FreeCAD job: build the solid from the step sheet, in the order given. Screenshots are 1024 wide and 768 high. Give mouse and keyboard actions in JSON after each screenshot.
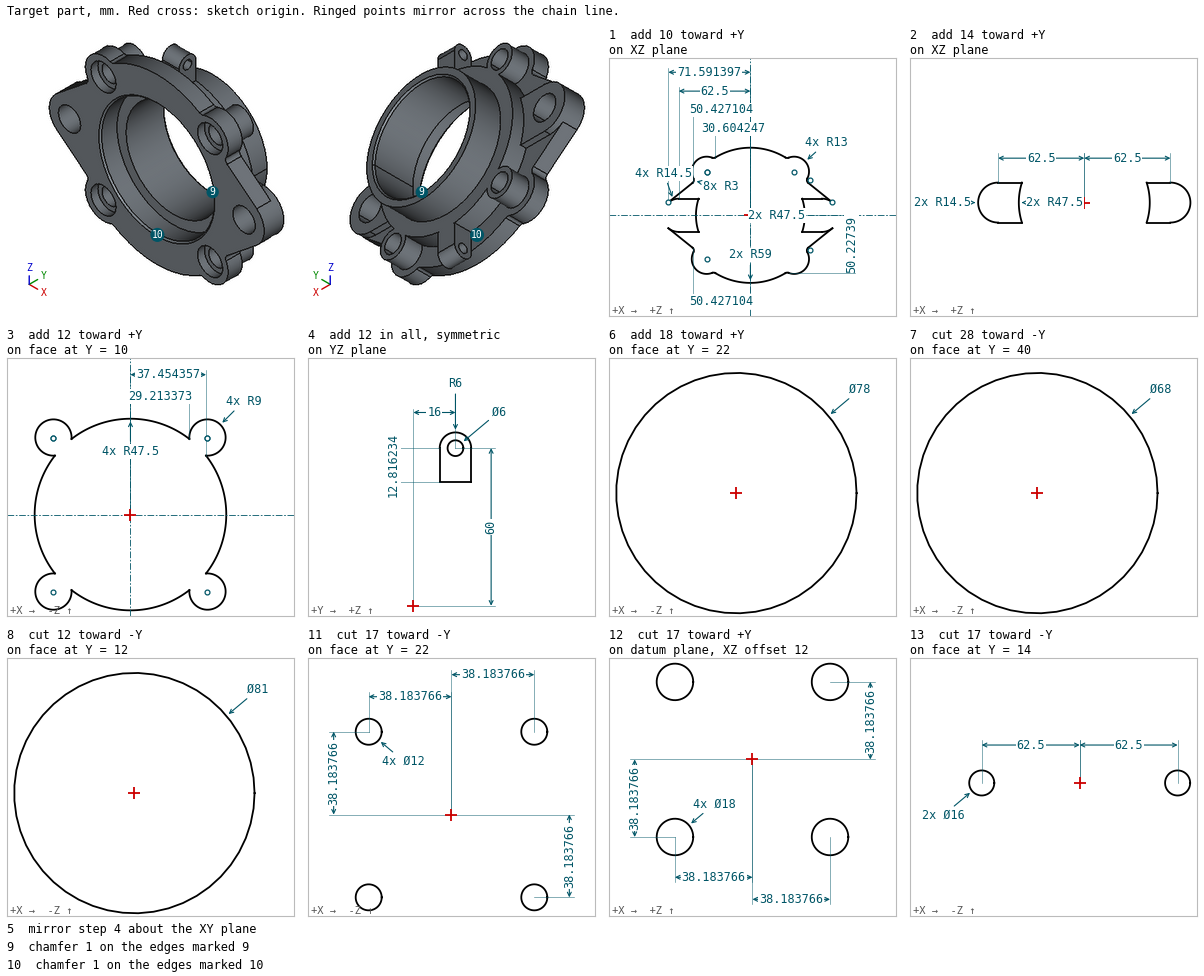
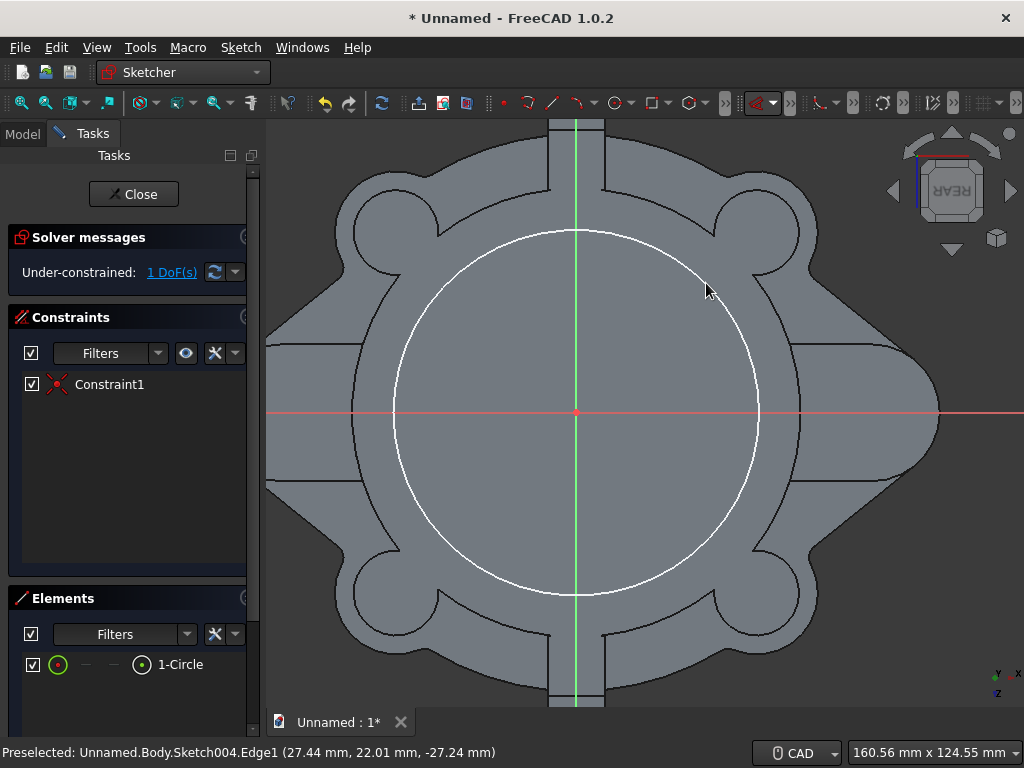
{"action": "key", "text": "d"}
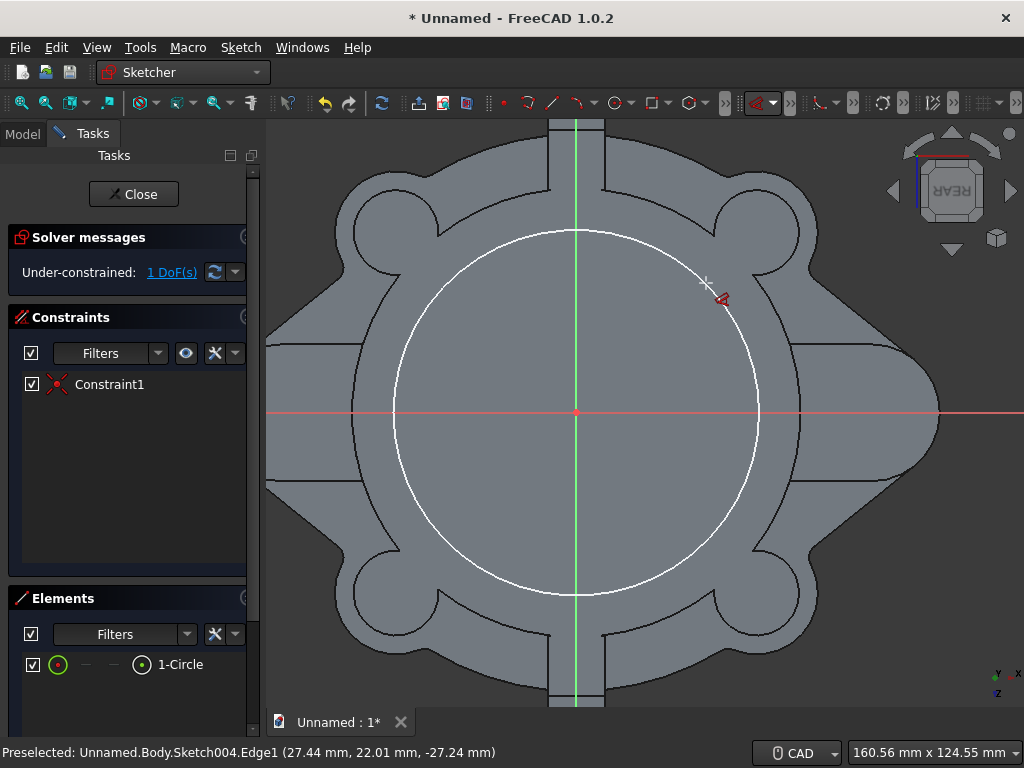
{"action": "left_click", "coordinate": [705, 283]}
{"action": "left_click", "coordinate": [728, 260]}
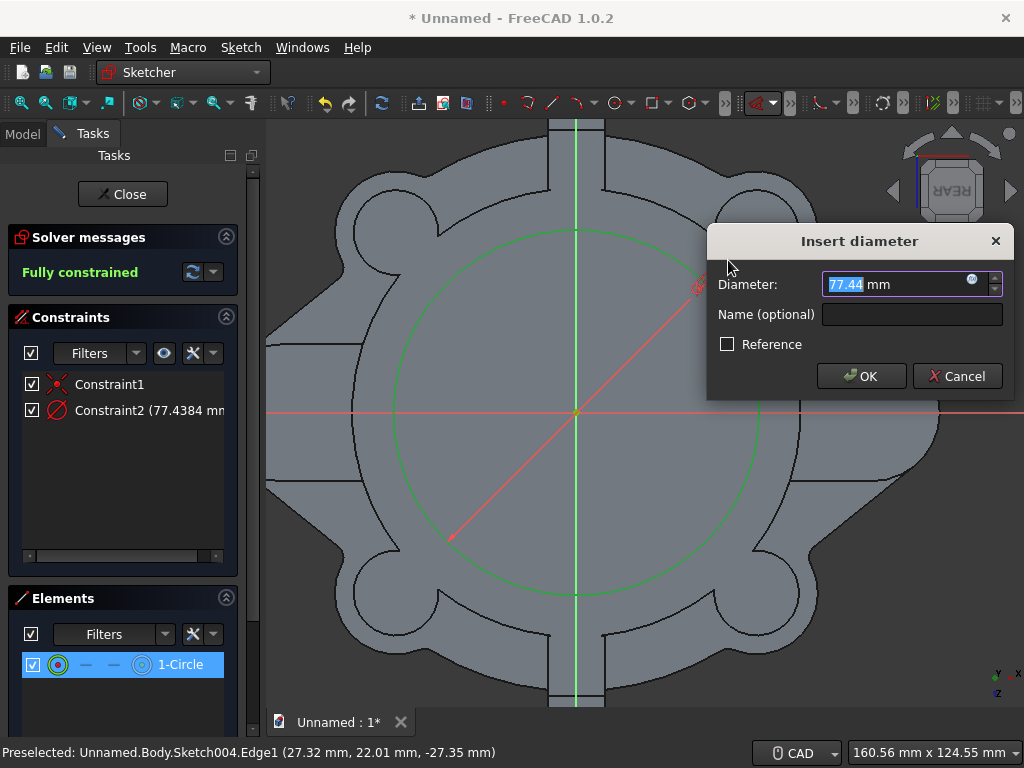
{"action": "type", "text": "78"}
{"action": "key", "text": "Return"}
{"action": "key", "text": "Escape"}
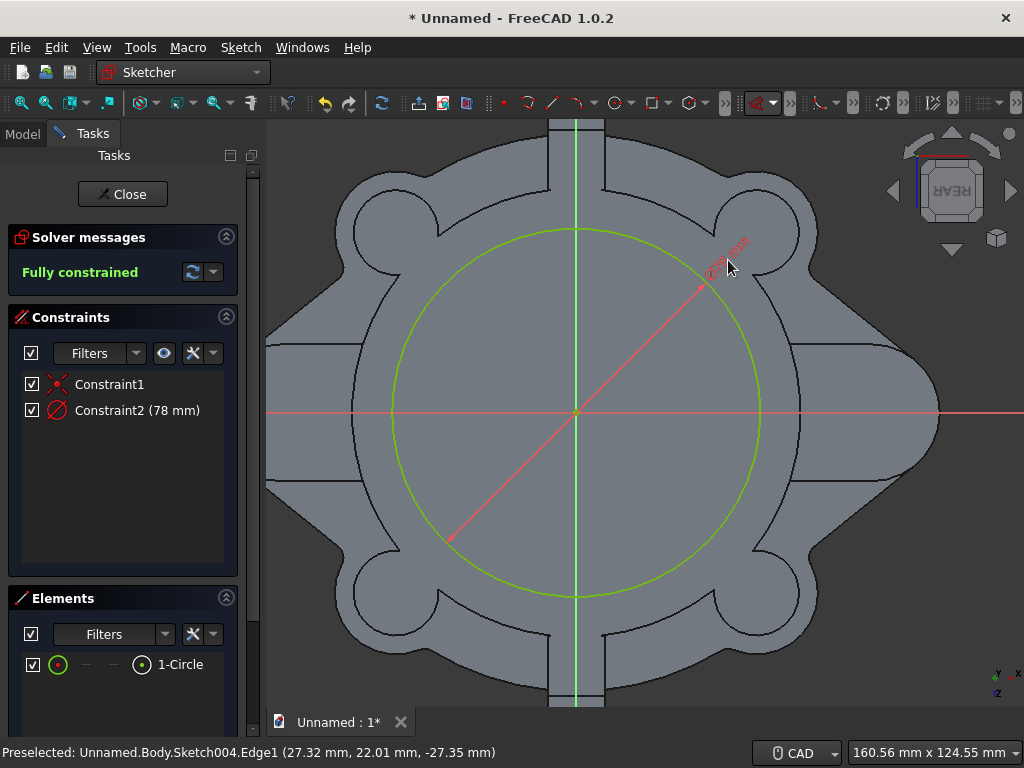
{"action": "left_click", "coordinate": [123, 194]}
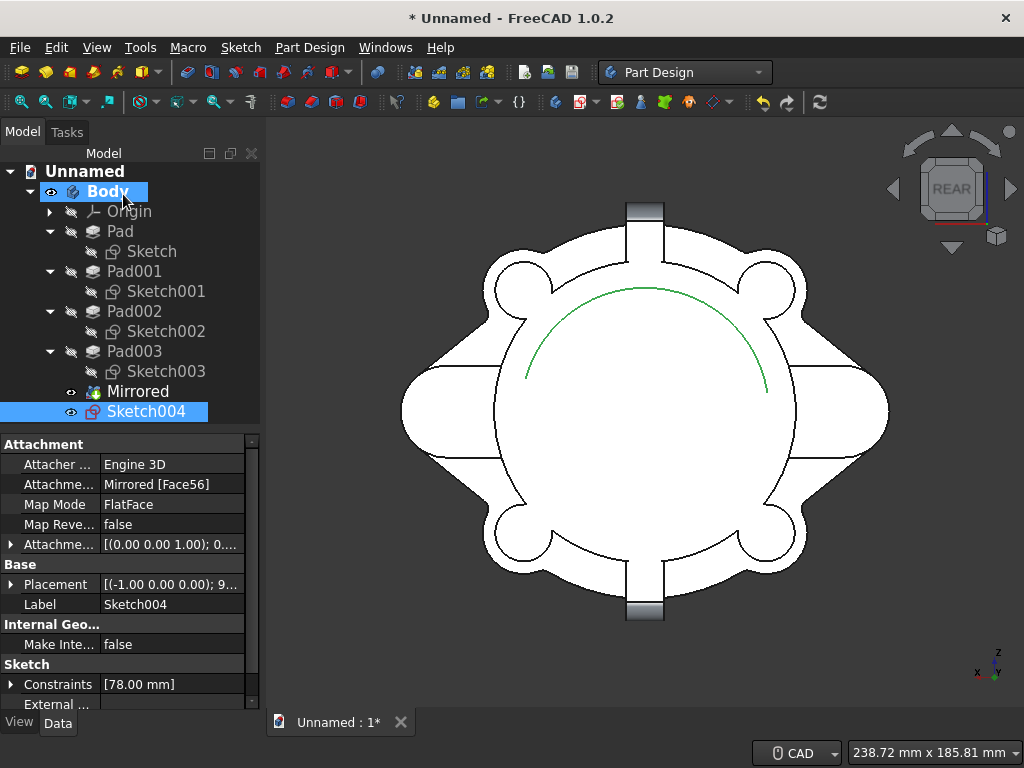
{"action": "left_click", "coordinate": [22, 72]}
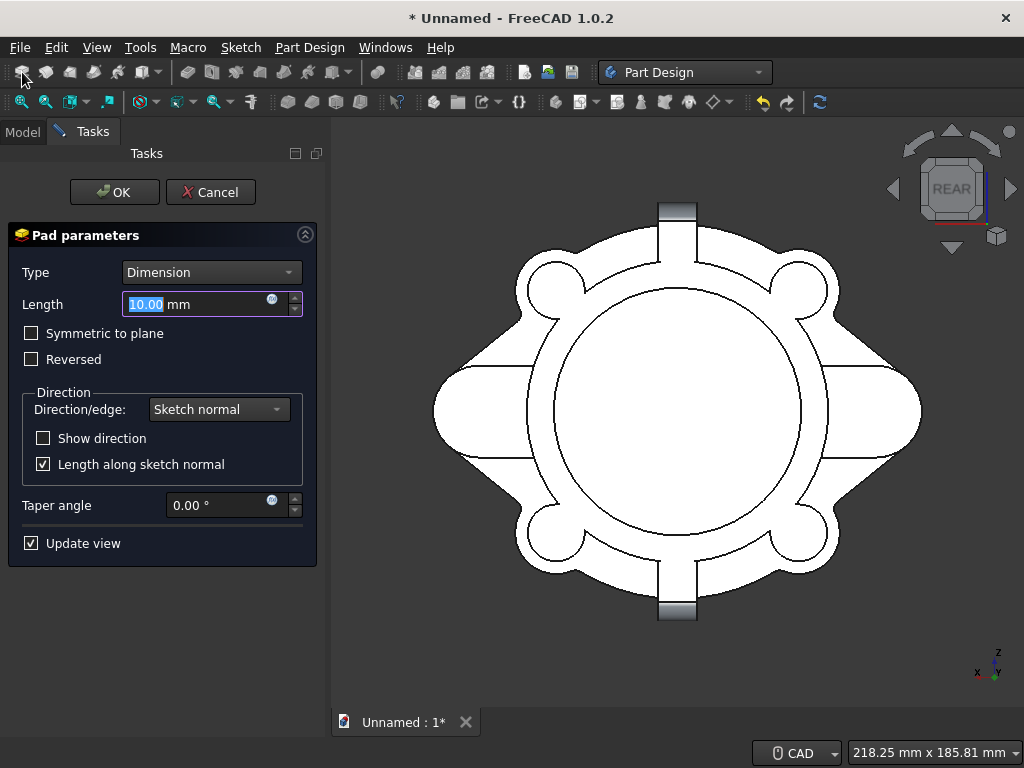
{"action": "type", "text": "18"}
{"action": "key", "text": "Tab"}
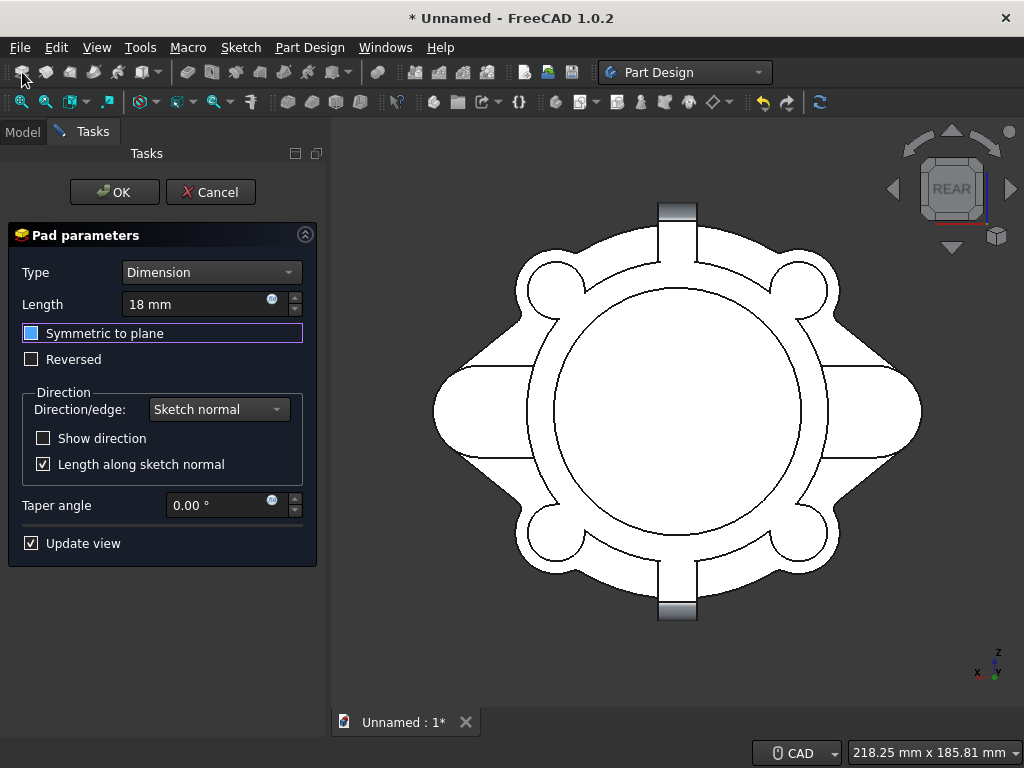
{"action": "left_click", "coordinate": [115, 192]}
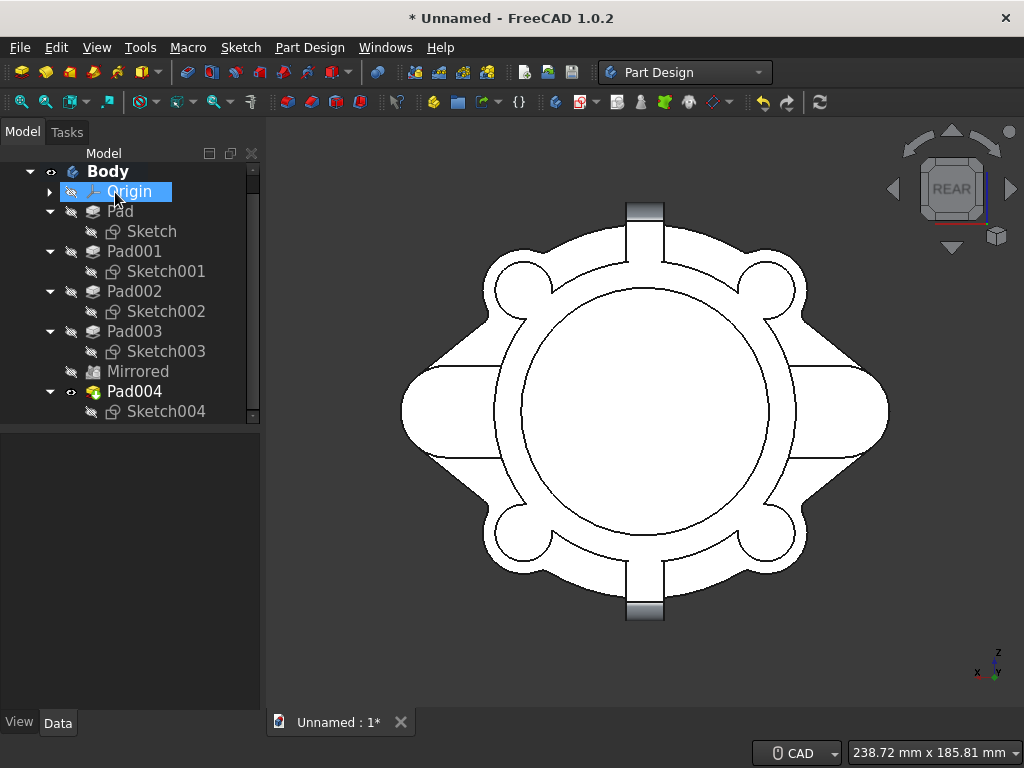
{"action": "left_click", "coordinate": [645, 411]}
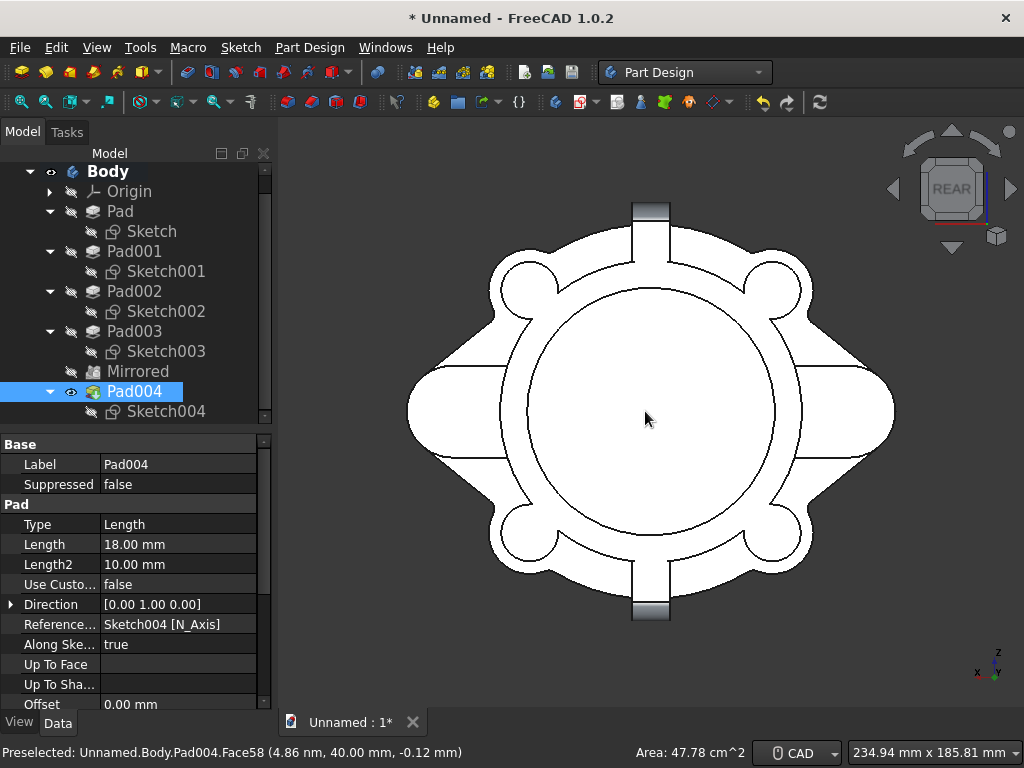
{"action": "left_click", "coordinate": [580, 102]}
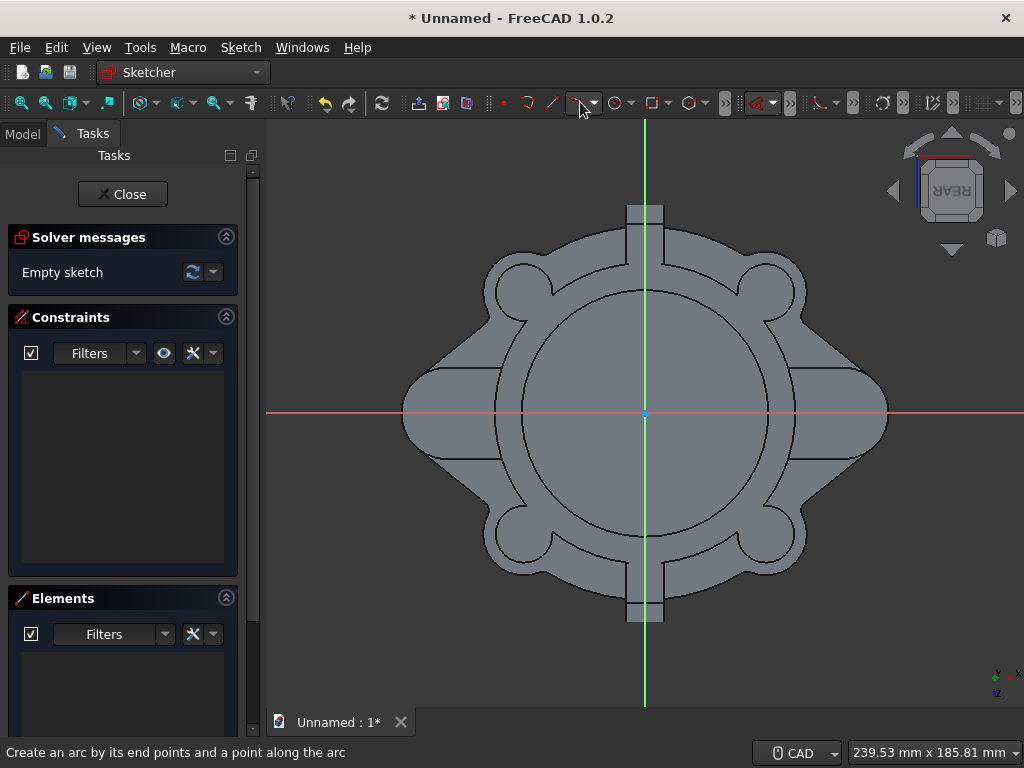
{"action": "scroll", "coordinate": [728, 414], "scroll_direction": "up", "scroll_amount": 3}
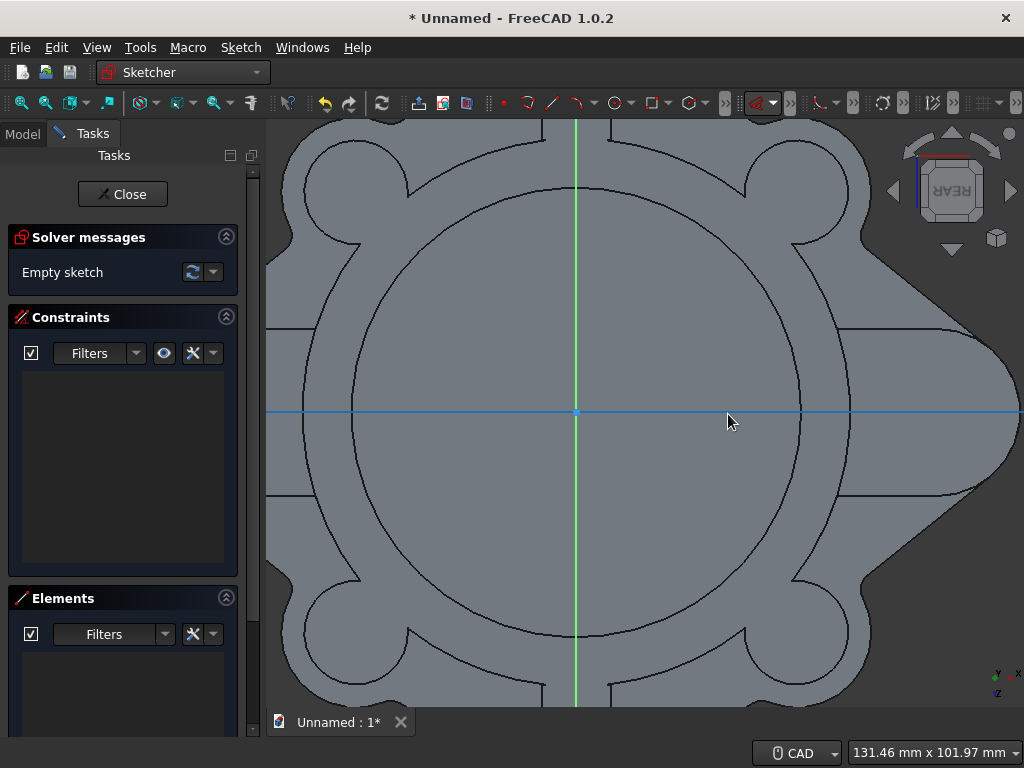
{"action": "left_click", "coordinate": [616, 104]}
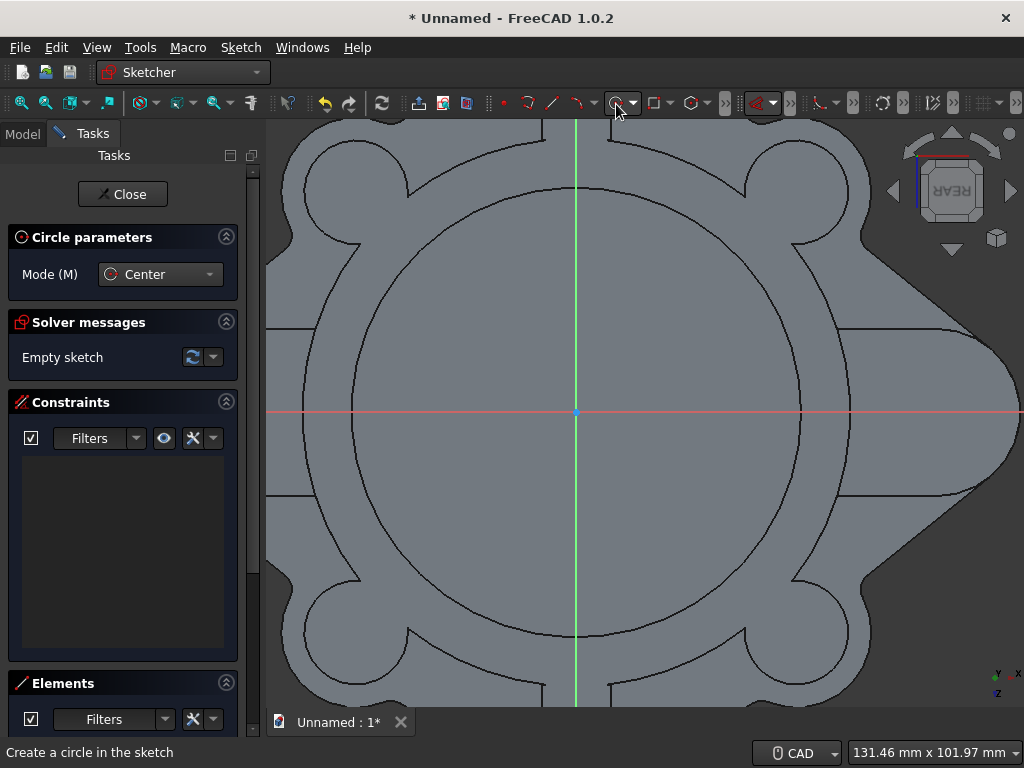
{"action": "left_click", "coordinate": [576, 412]}
{"action": "left_click", "coordinate": [715, 274]}
{"action": "key", "text": "Escape"}